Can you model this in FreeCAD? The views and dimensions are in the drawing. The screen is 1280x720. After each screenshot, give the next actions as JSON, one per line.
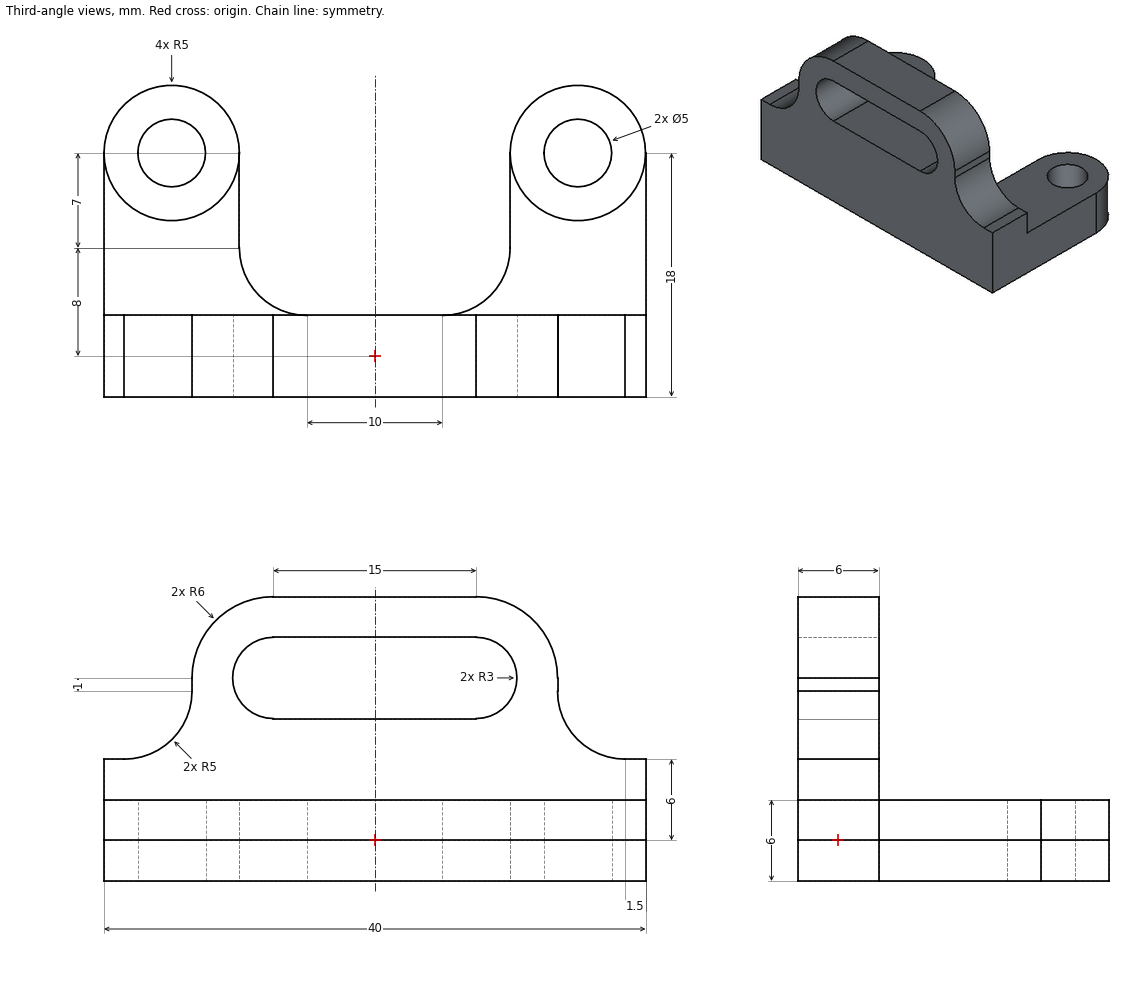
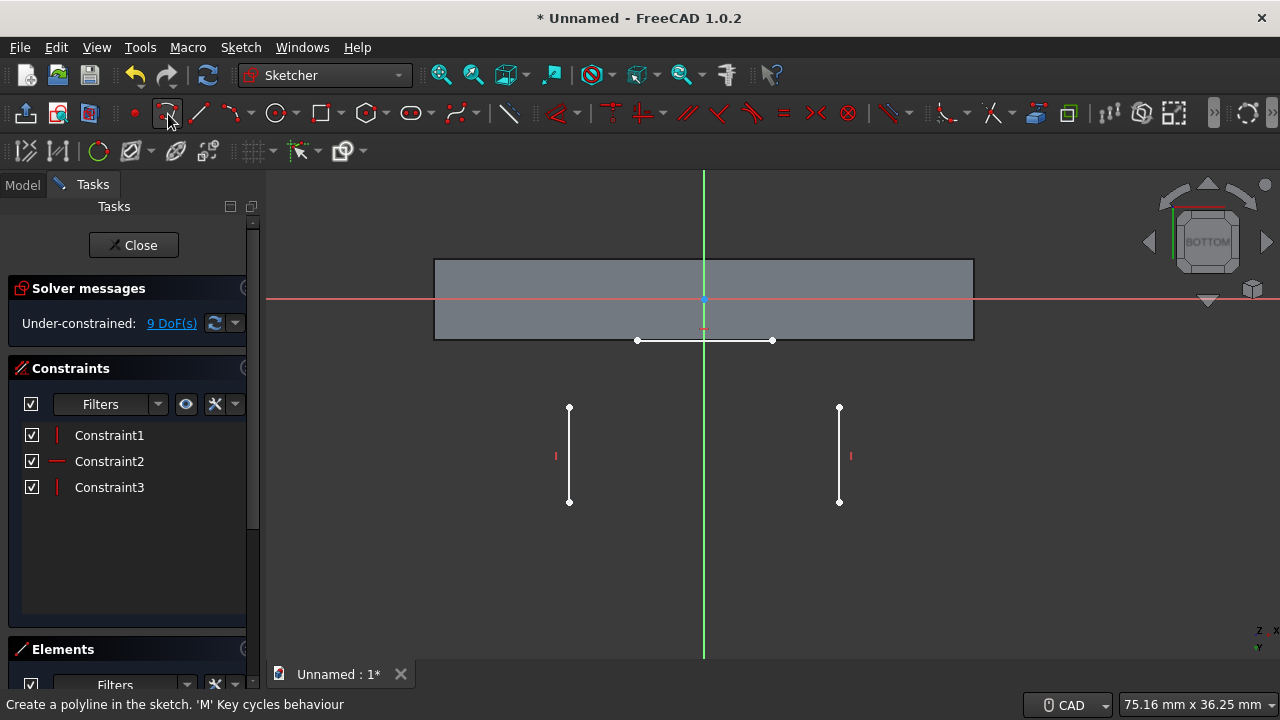
{"action": "left_click", "coordinate": [974, 502]}
{"action": "left_click", "coordinate": [974, 259]}
{"action": "left_click", "coordinate": [434, 259]}
{"action": "left_click", "coordinate": [434, 502]}
{"action": "right_click", "coordinate": [434, 502]}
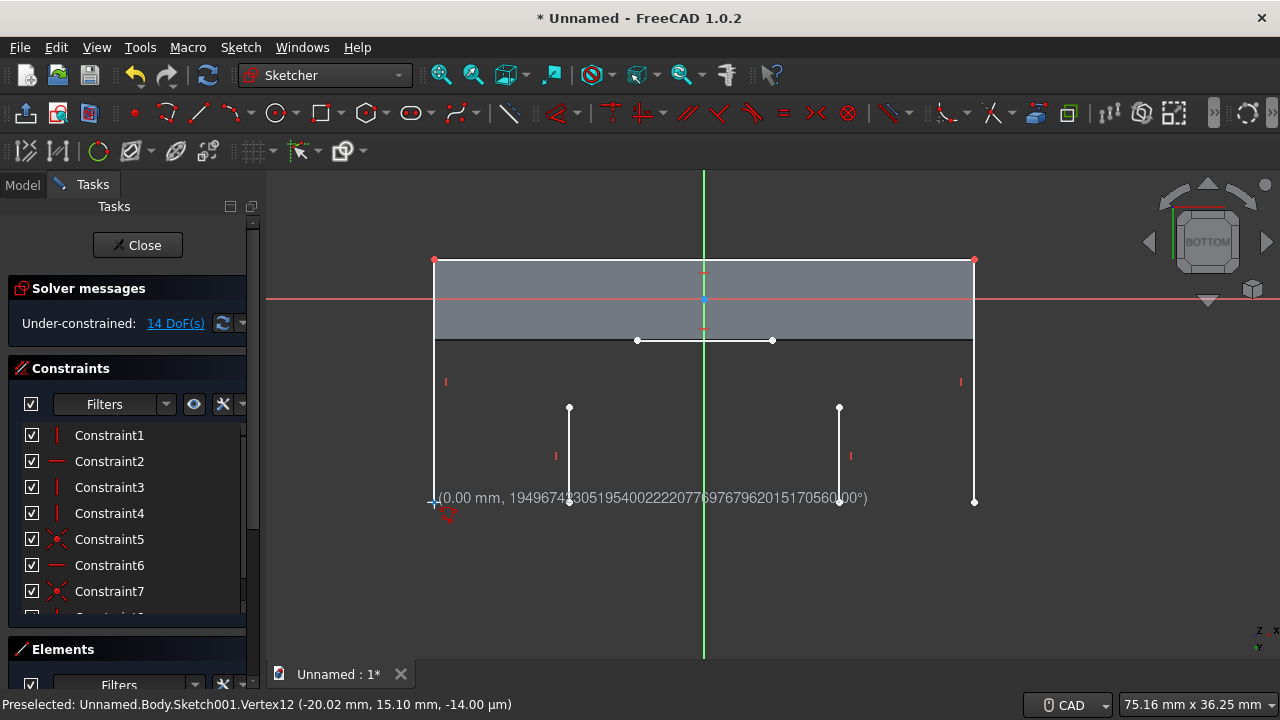
{"action": "left_click", "coordinate": [232, 114]}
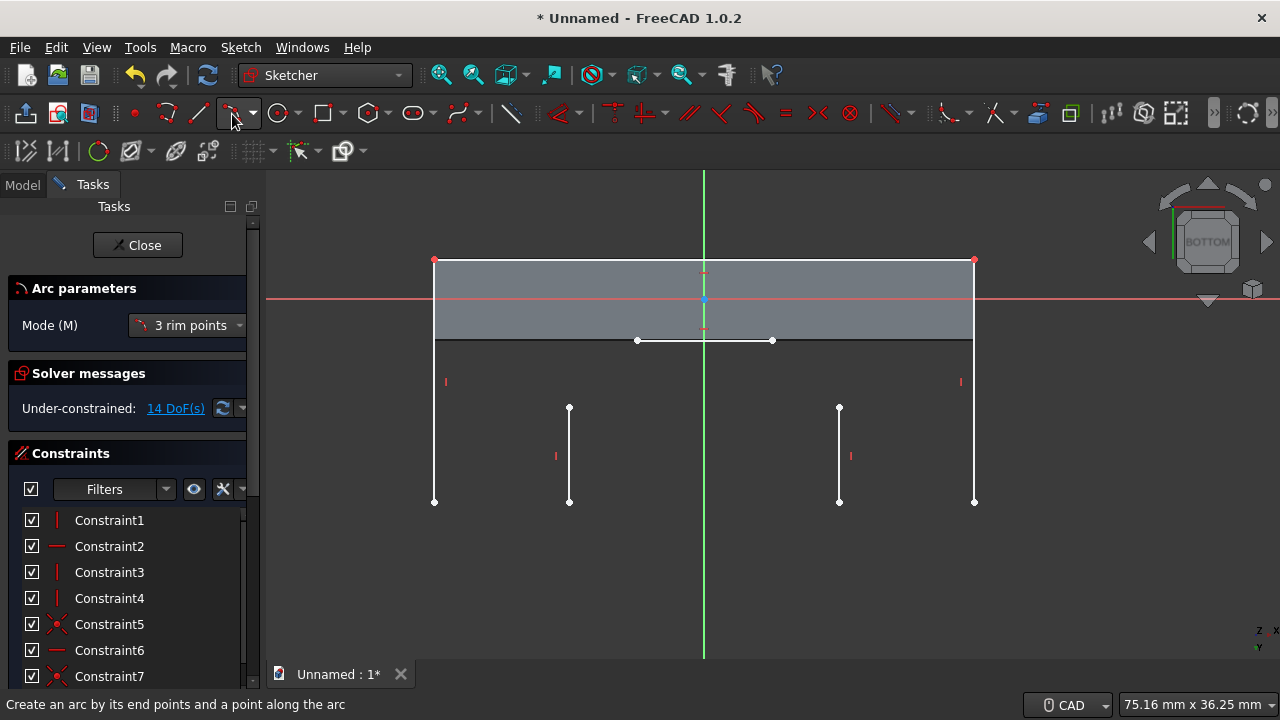
{"action": "left_click", "coordinate": [569, 408]}
{"action": "left_click", "coordinate": [637, 341]}
{"action": "left_click", "coordinate": [589, 360]}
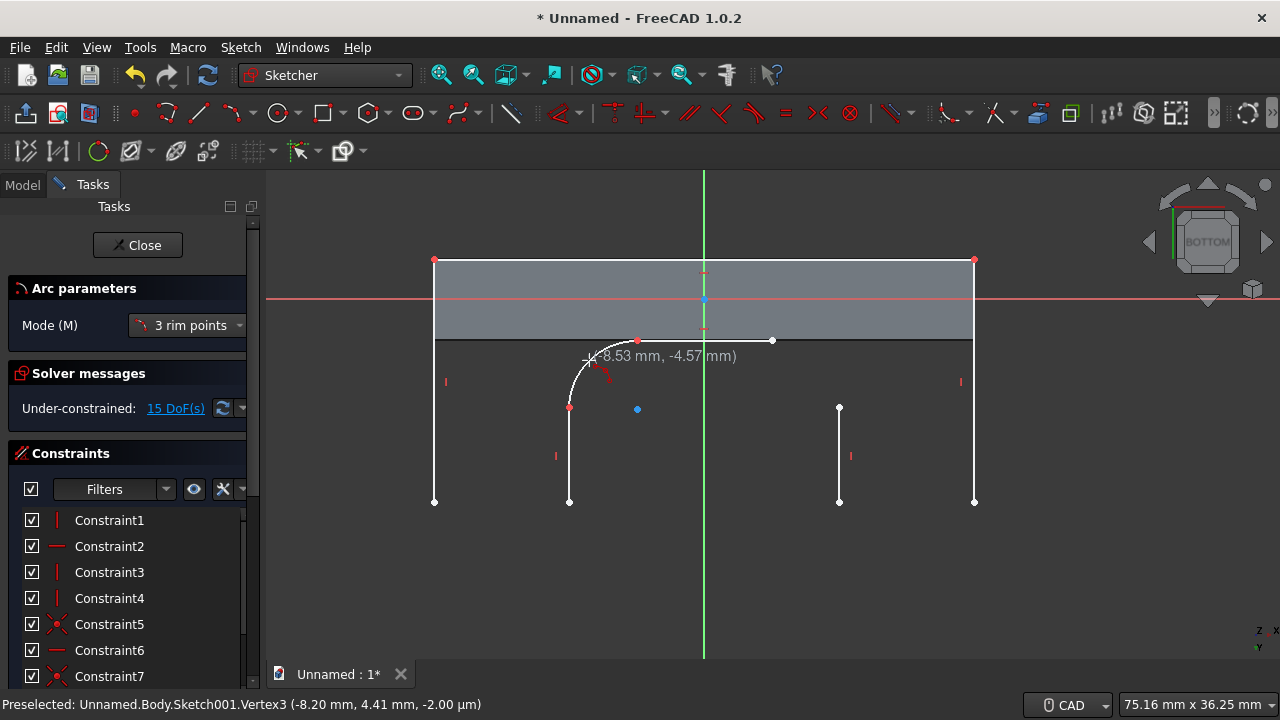
{"action": "left_click", "coordinate": [772, 341]}
{"action": "left_click", "coordinate": [839, 408]}
{"action": "left_click", "coordinate": [819, 360]}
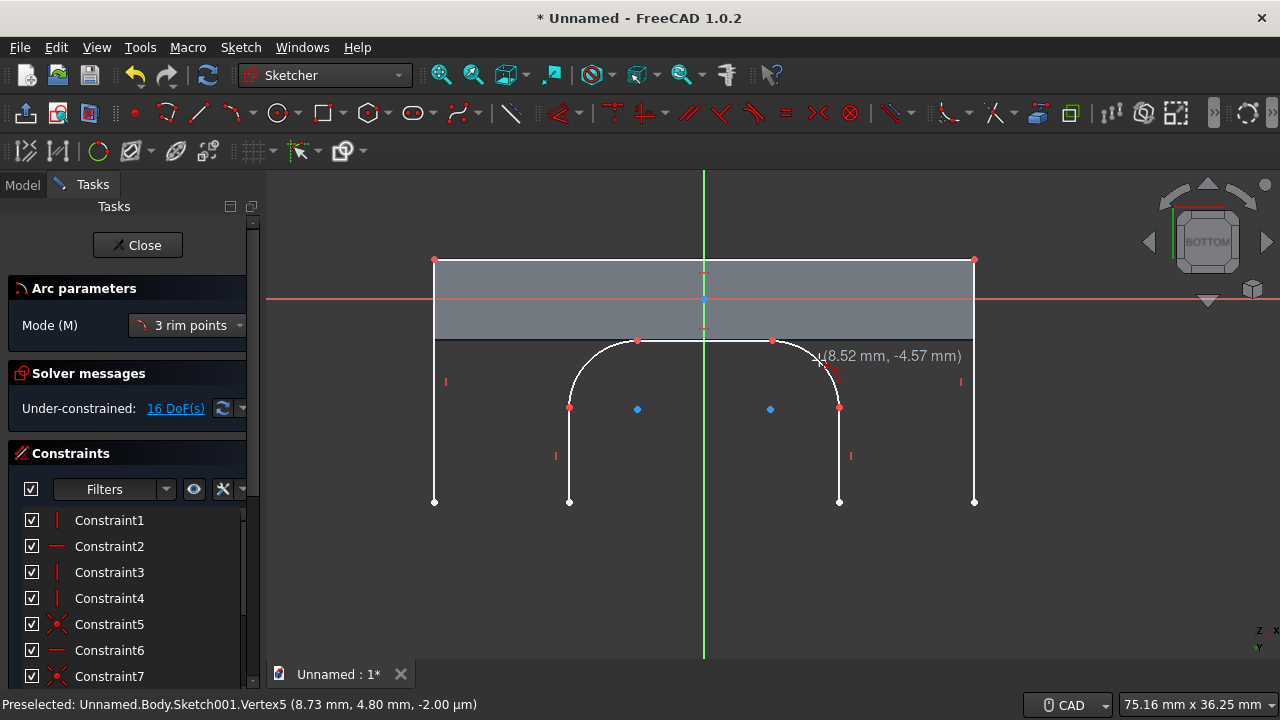
{"action": "left_click", "coordinate": [839, 503]}
{"action": "left_click", "coordinate": [974, 503]}
{"action": "left_click", "coordinate": [906, 569]}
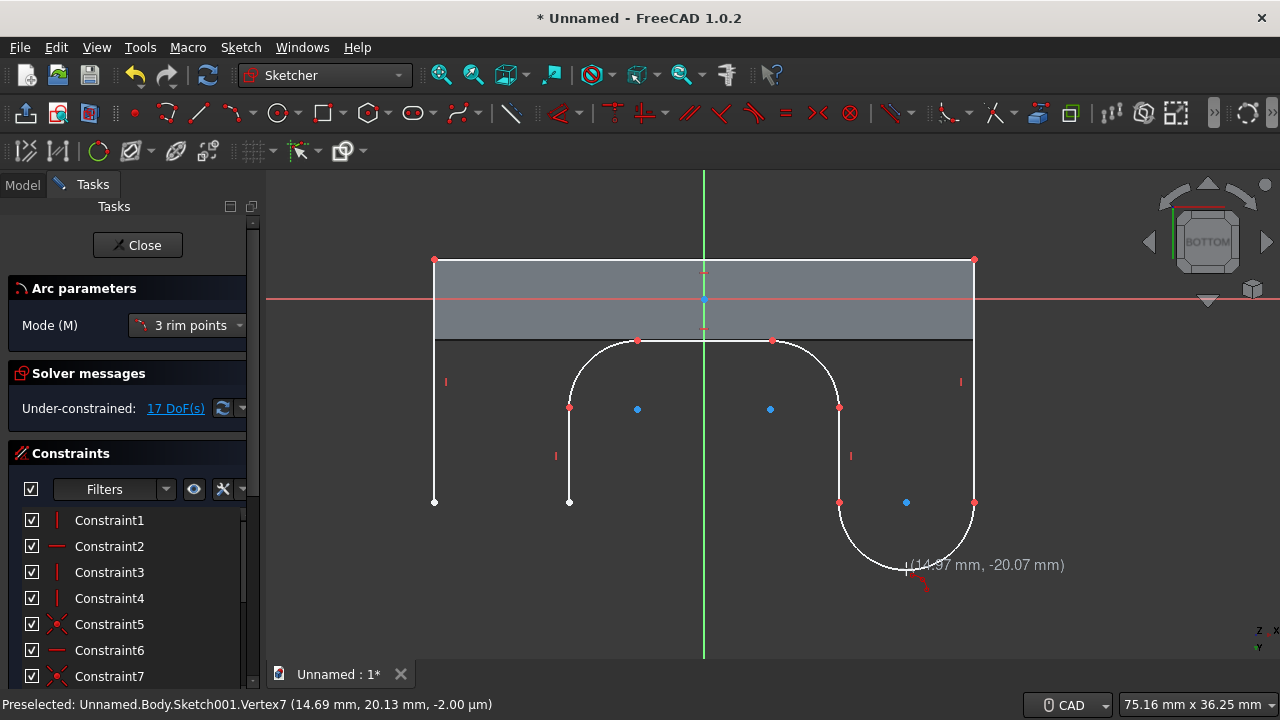
{"action": "left_click", "coordinate": [434, 503]}
{"action": "left_click", "coordinate": [569, 503]}
{"action": "left_click", "coordinate": [502, 569]}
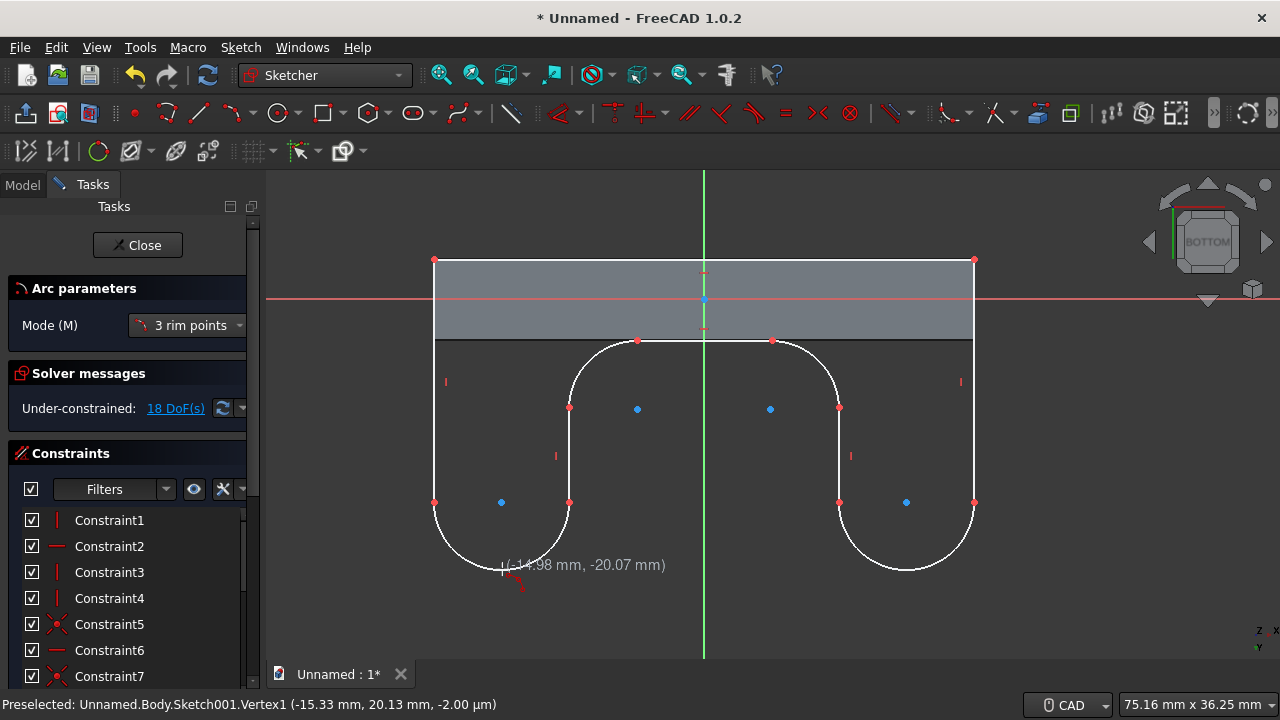
{"action": "key", "text": "g c"}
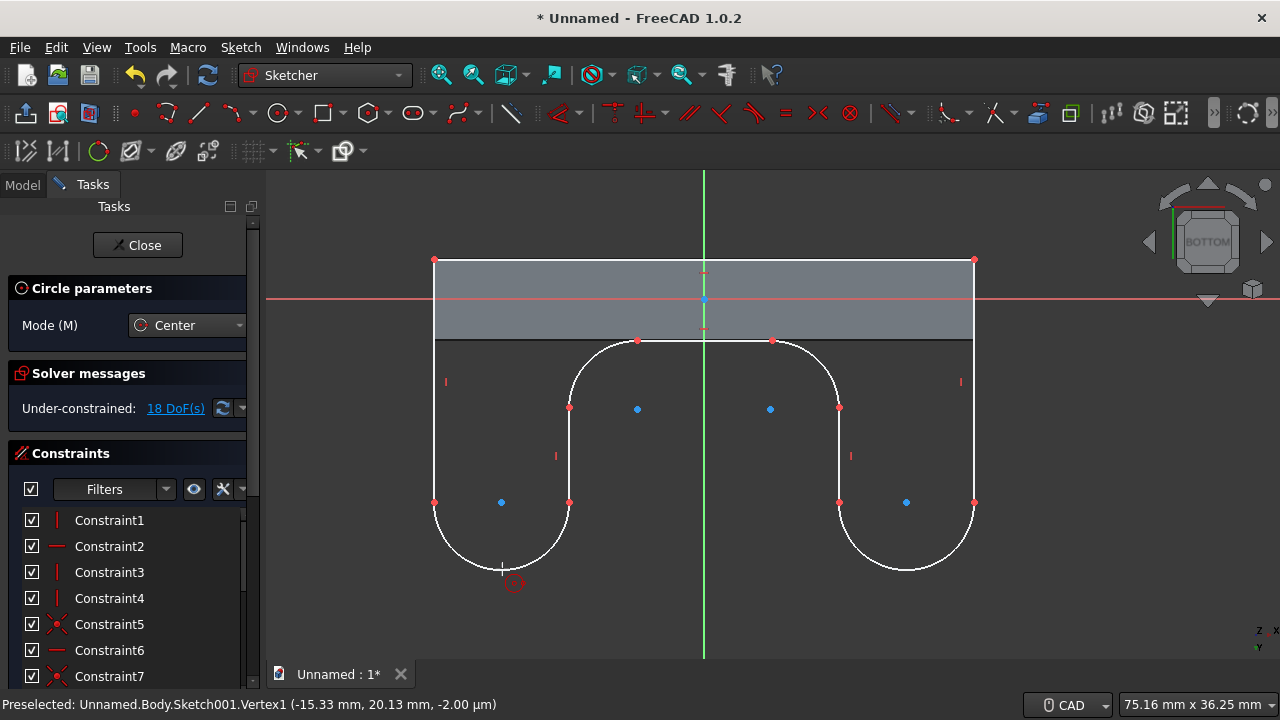
{"action": "left_click", "coordinate": [906, 502]}
{"action": "left_click", "coordinate": [930, 478]}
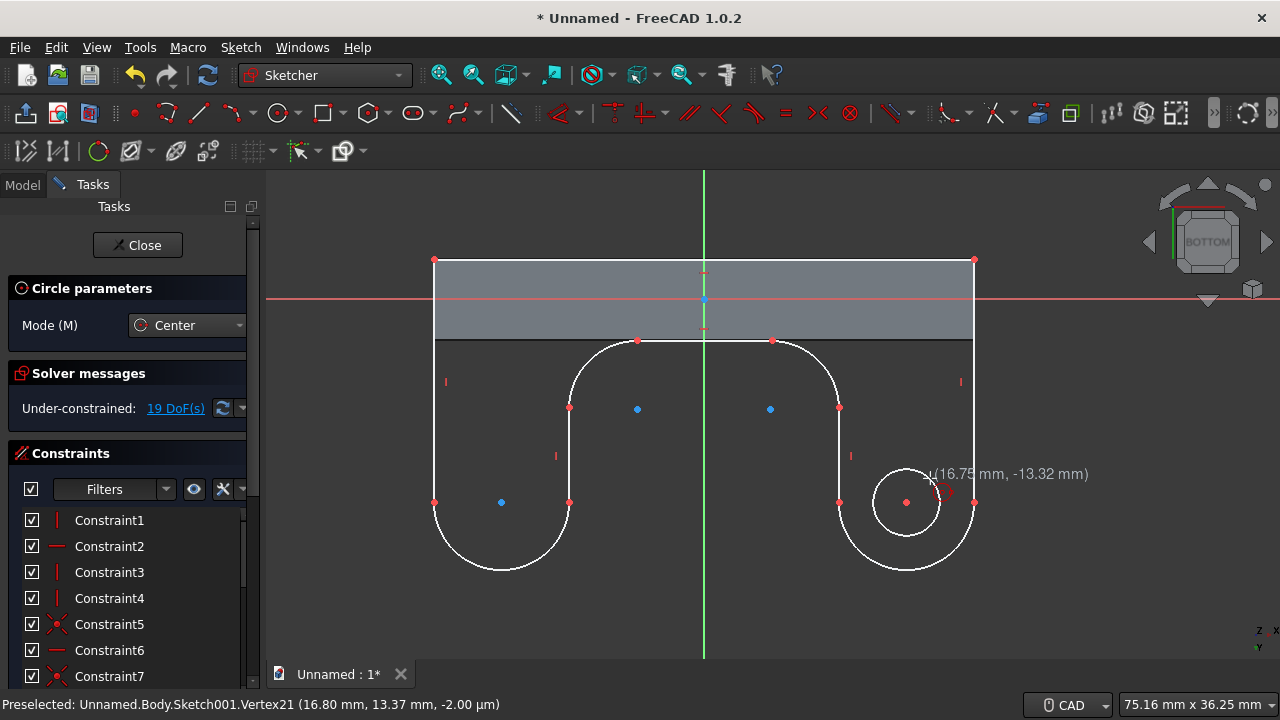
{"action": "left_click", "coordinate": [502, 502]}
{"action": "left_click", "coordinate": [526, 478]}
{"action": "key", "text": "Escape"}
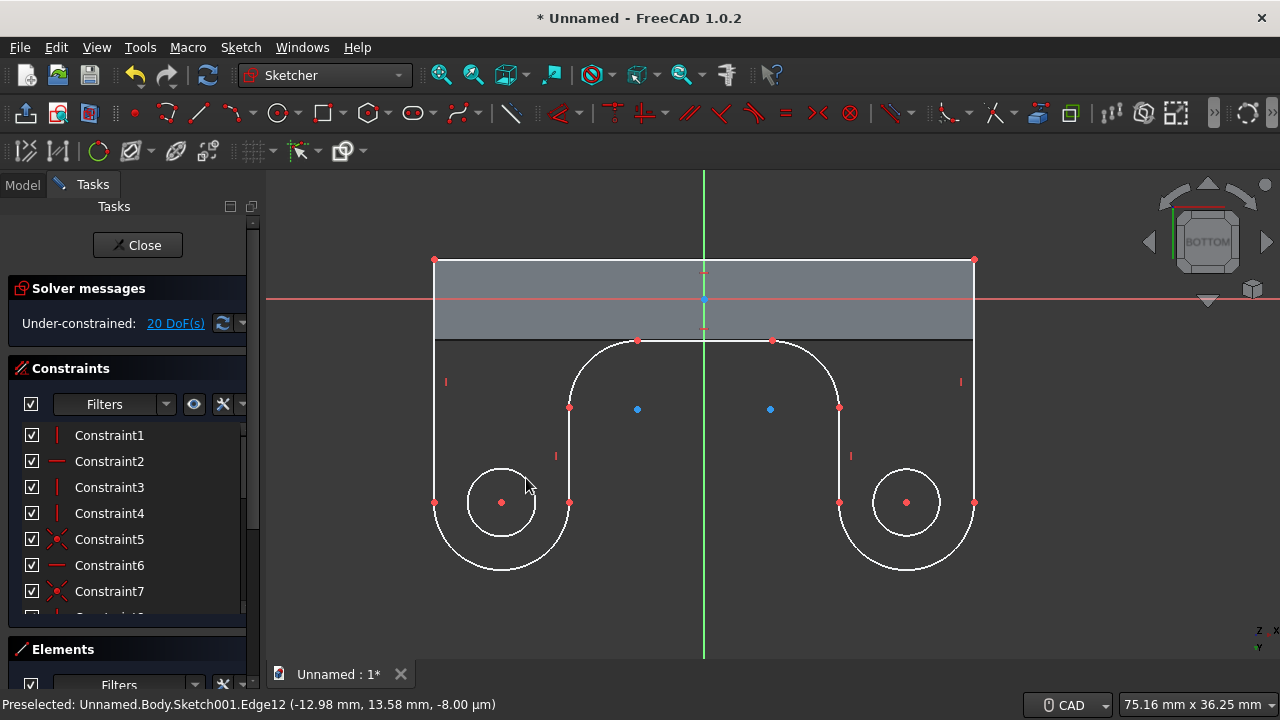
{"action": "left_click", "coordinate": [569, 475]}